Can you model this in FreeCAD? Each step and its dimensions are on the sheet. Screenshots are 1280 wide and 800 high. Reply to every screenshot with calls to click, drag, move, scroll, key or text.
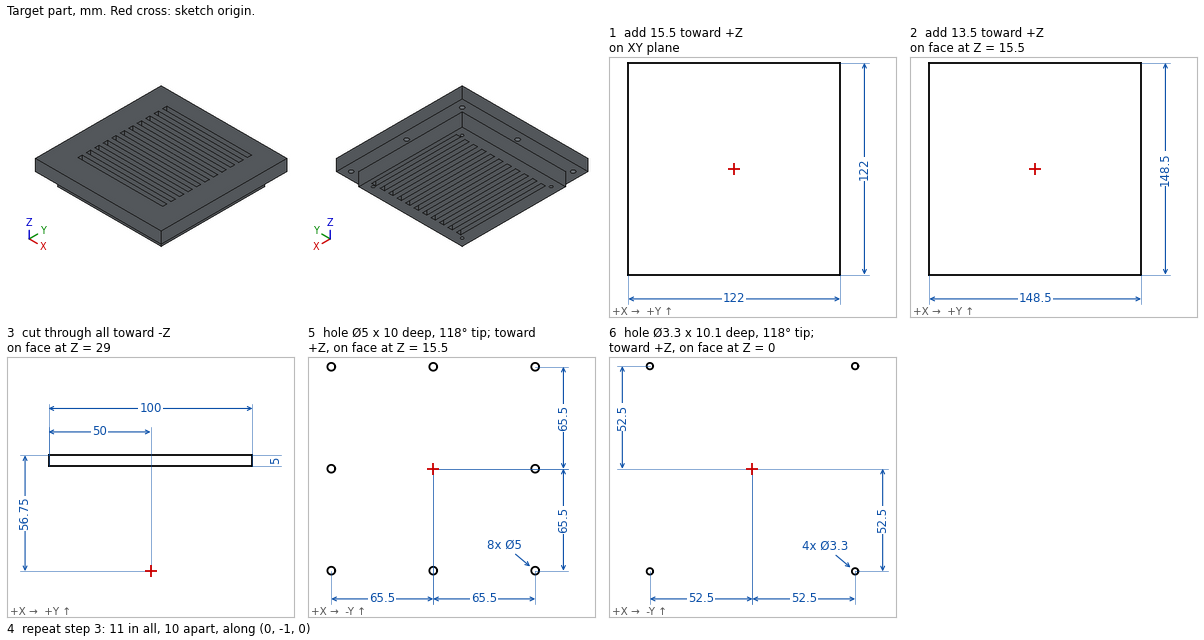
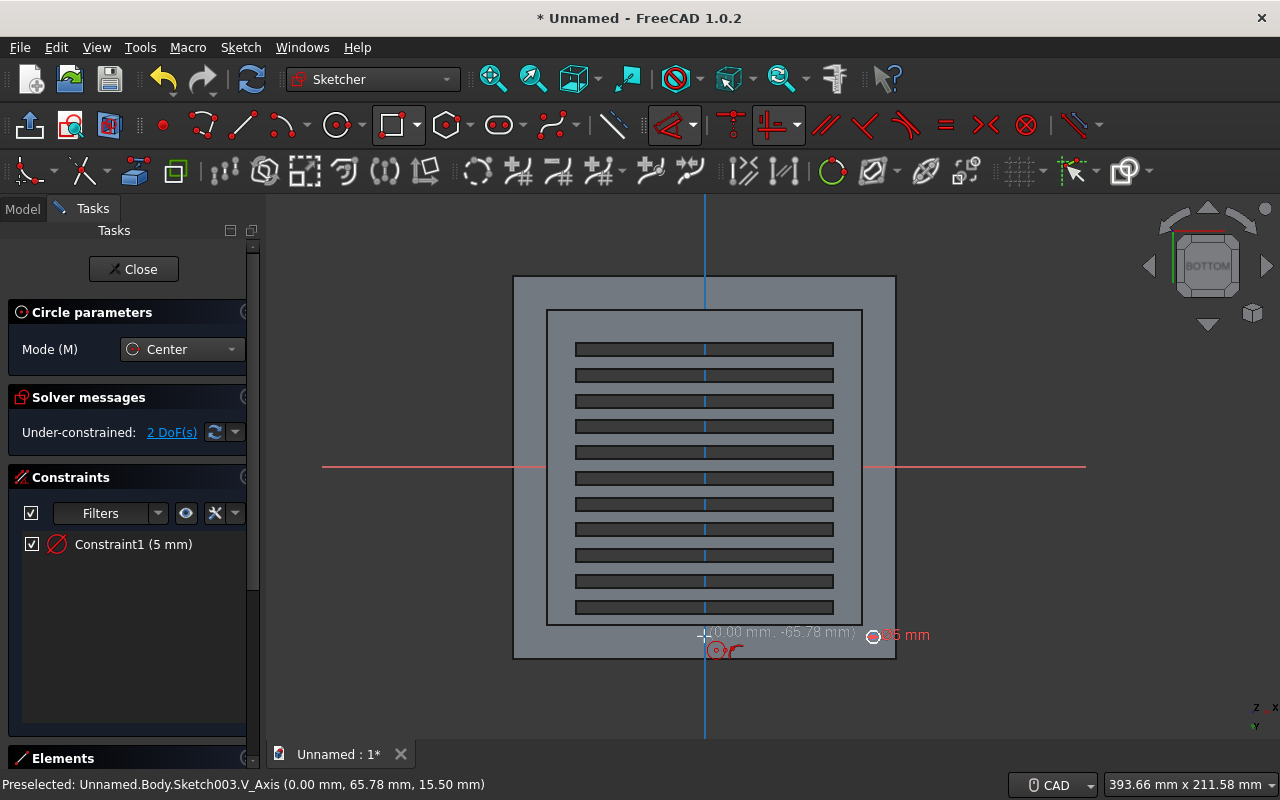
click(705, 636)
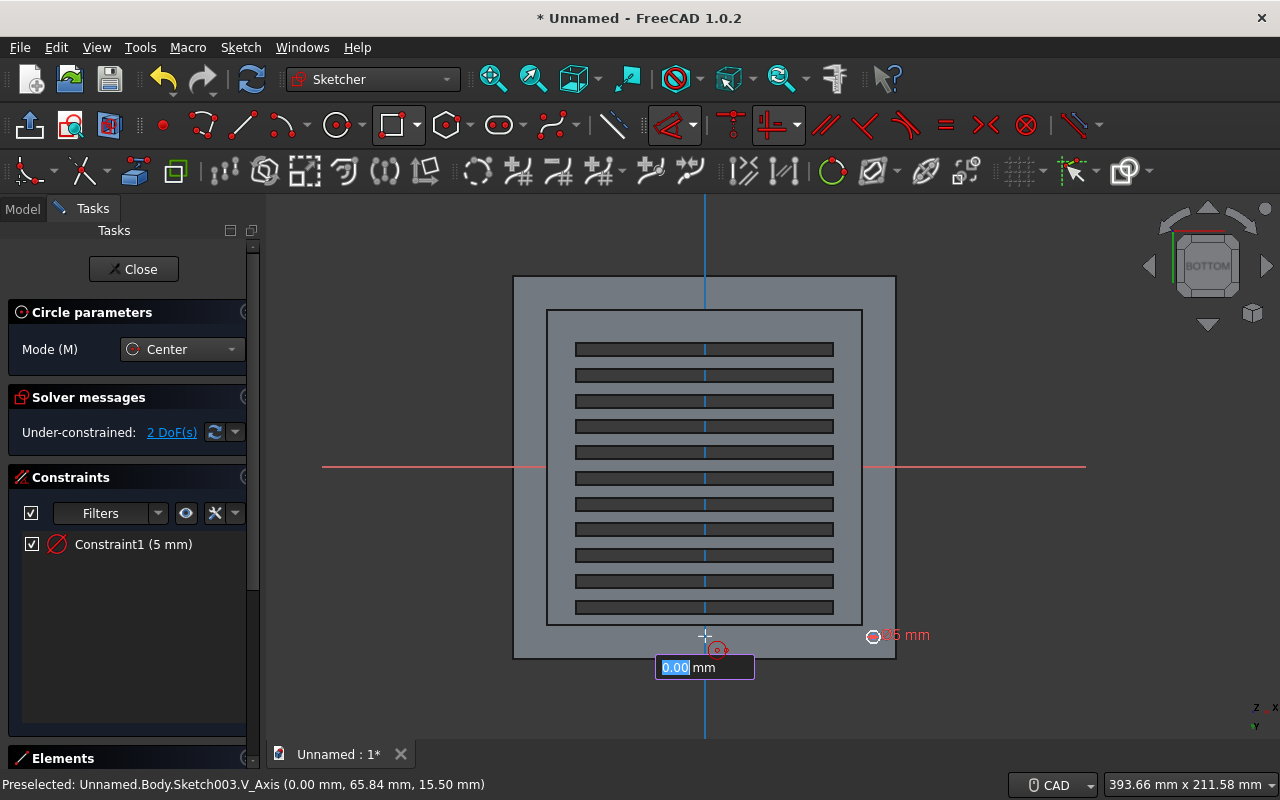
scroll(711, 634, up, 5)
move(709, 632)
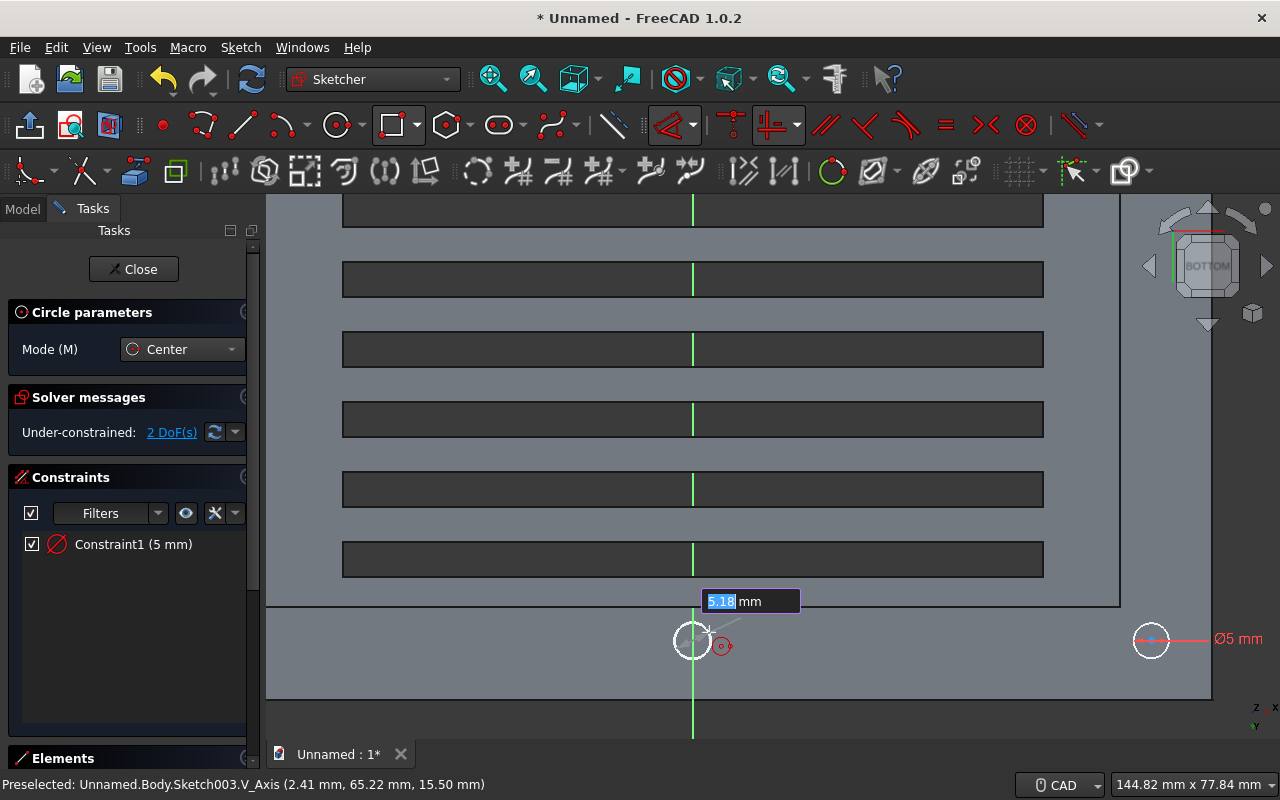
text(5)
key(Return)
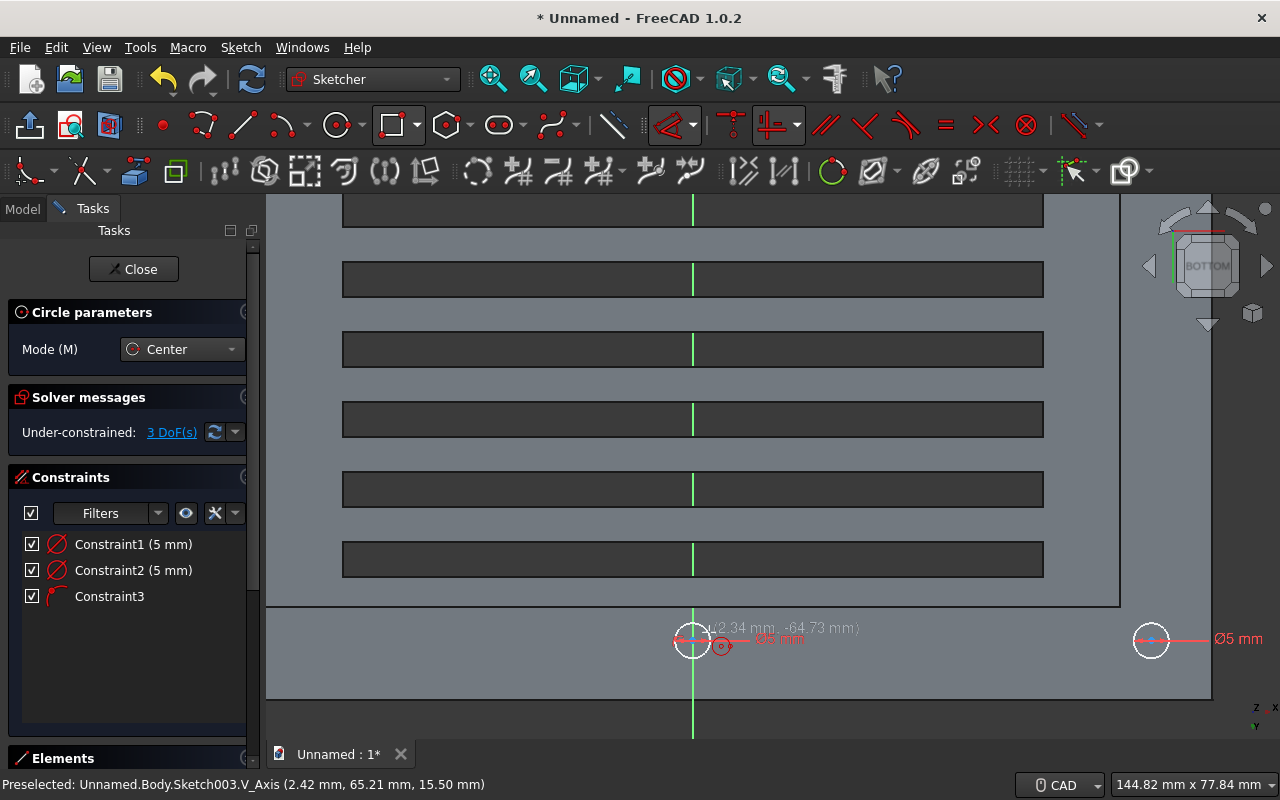
scroll(711, 633, down, 5)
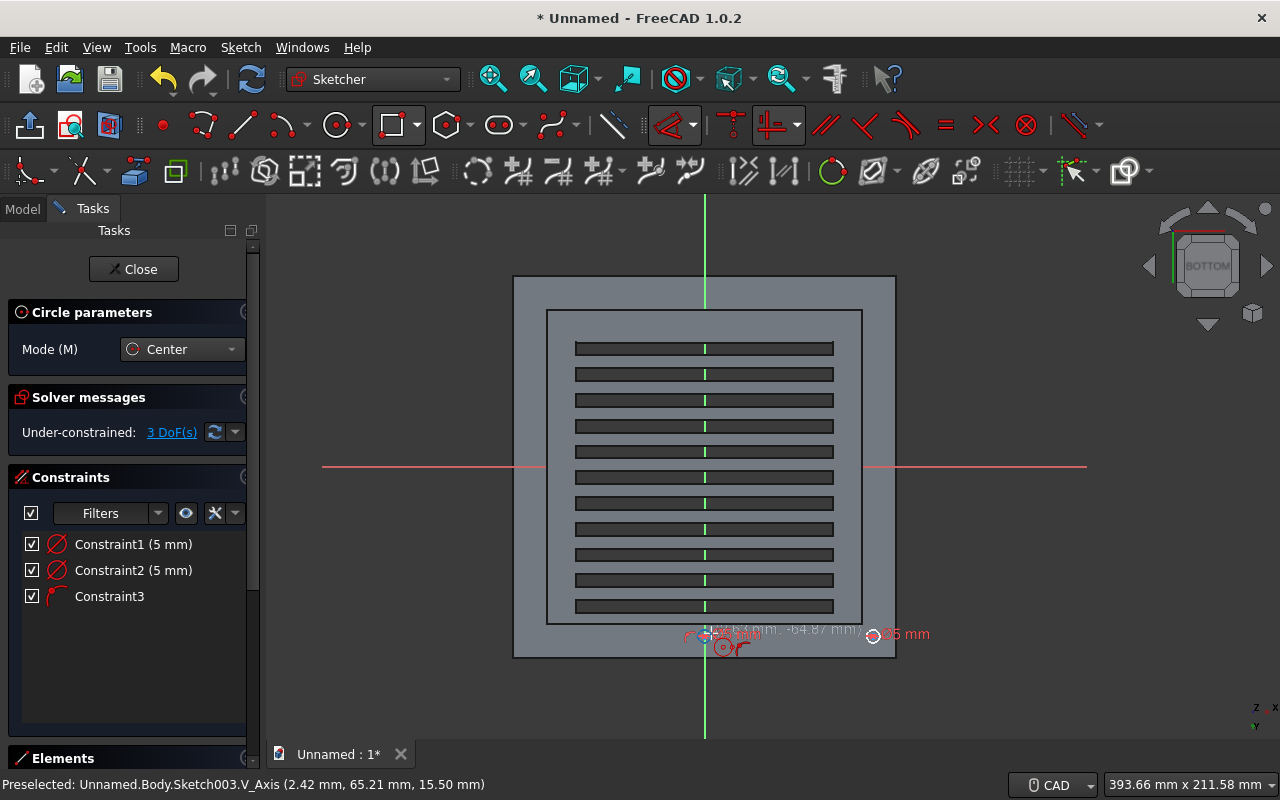
scroll(536, 636, up, 7)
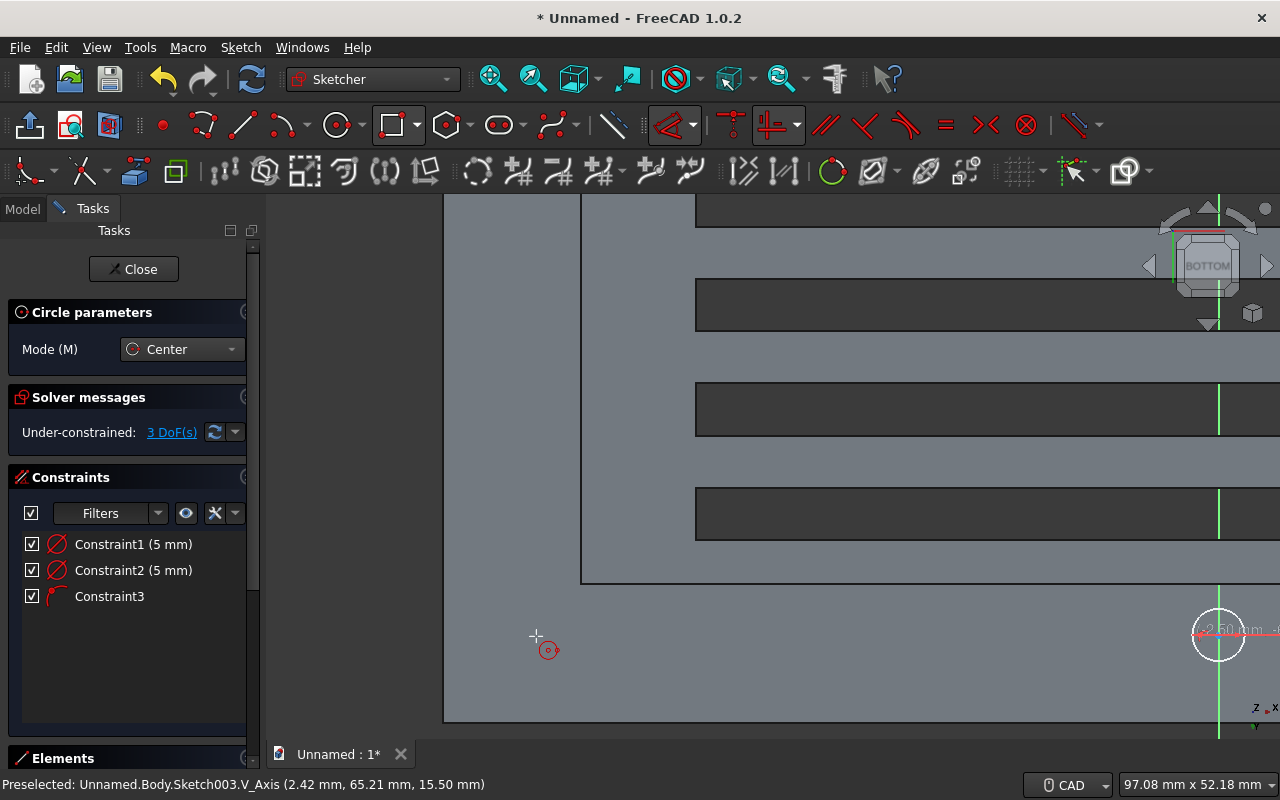
scroll(536, 636, down, 7)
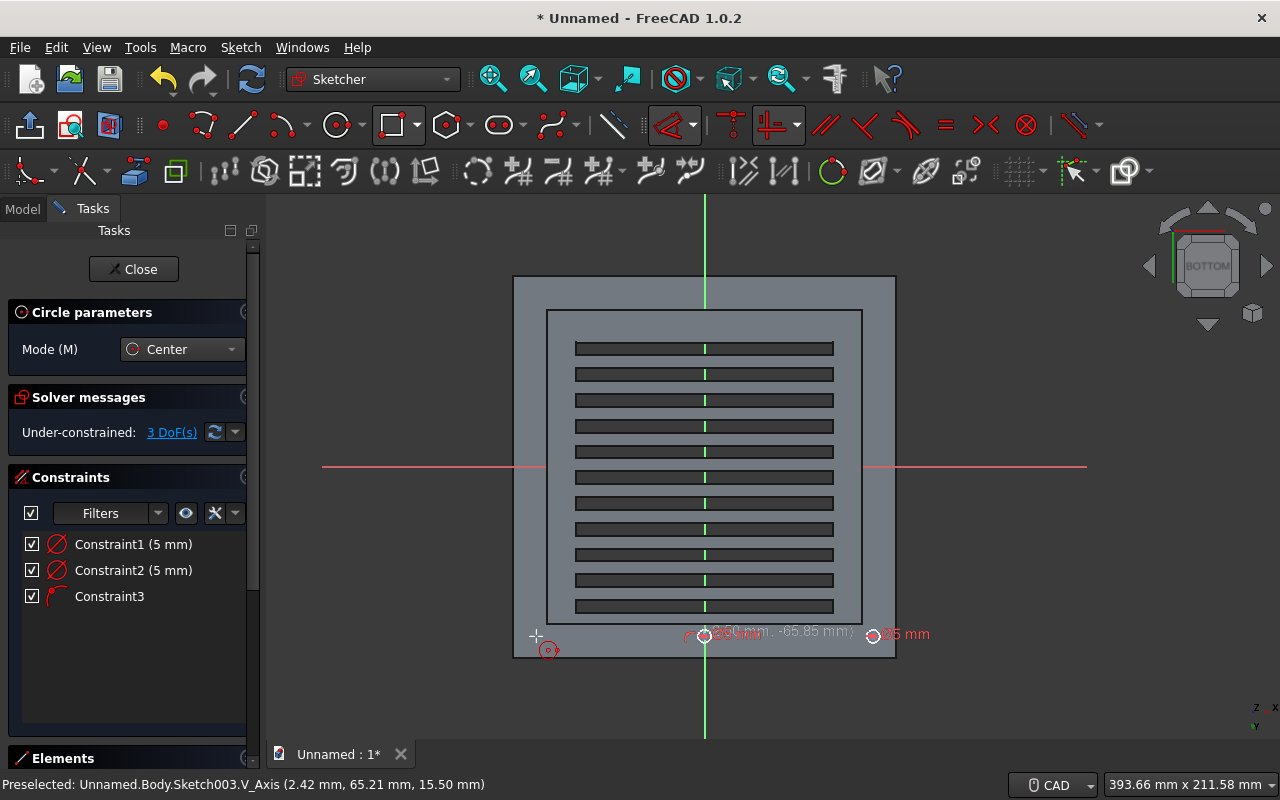
click(536, 636)
move(540, 631)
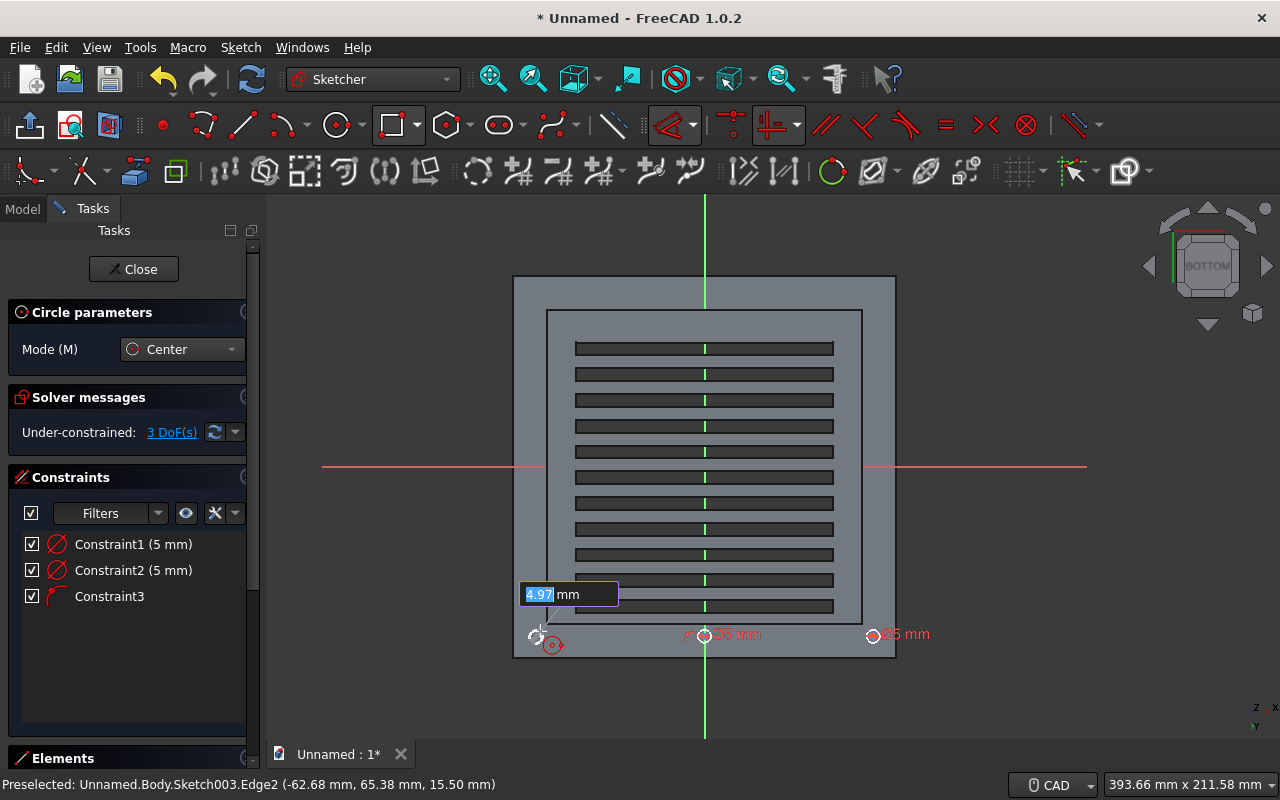
text(5)
key(Return)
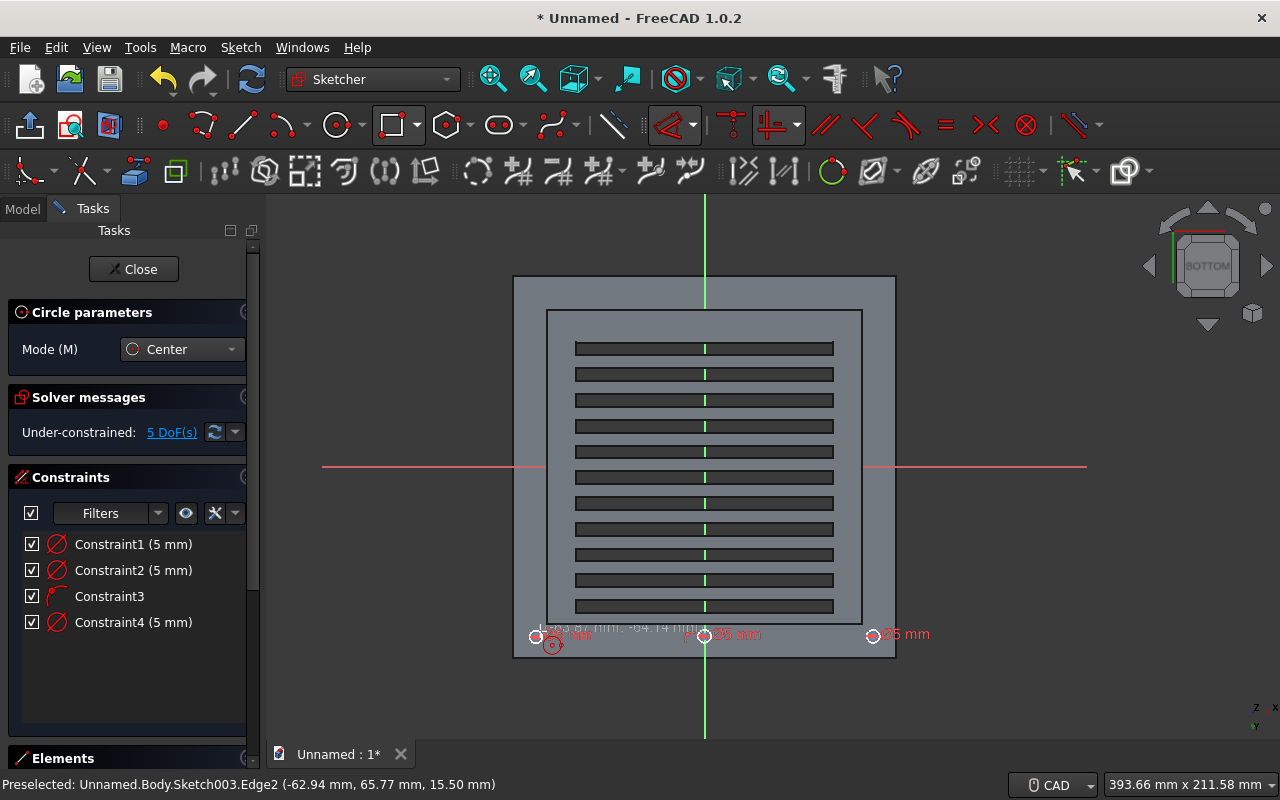
scroll(536, 467, up, 7)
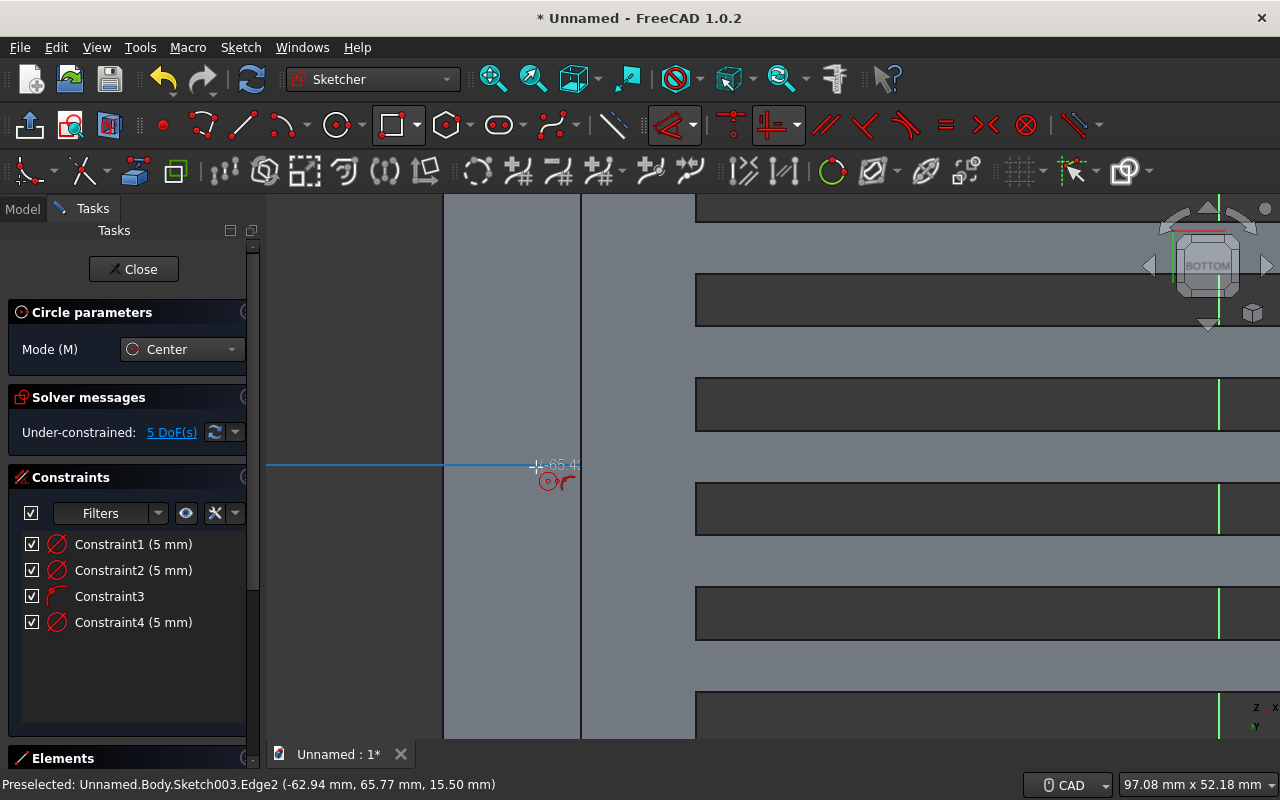
scroll(536, 467, down, 7)